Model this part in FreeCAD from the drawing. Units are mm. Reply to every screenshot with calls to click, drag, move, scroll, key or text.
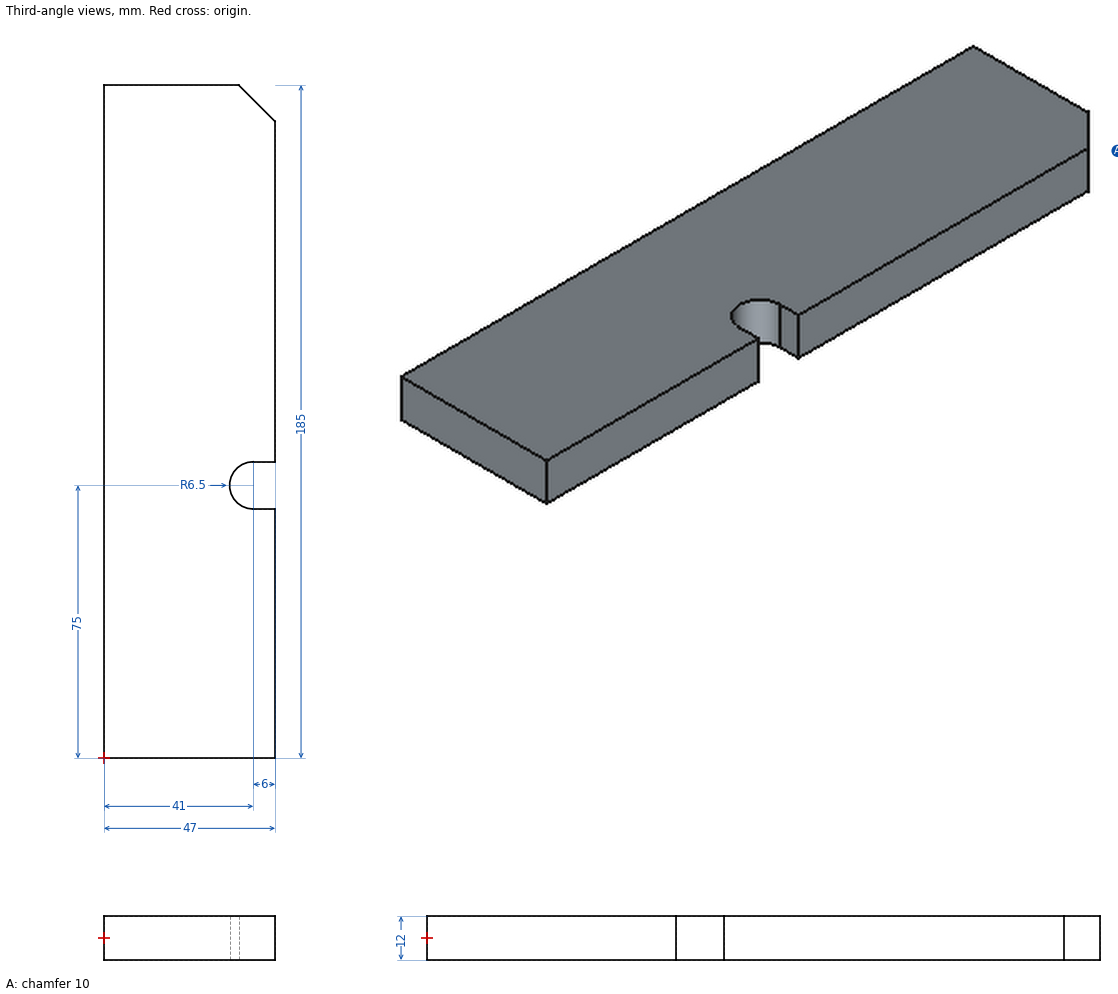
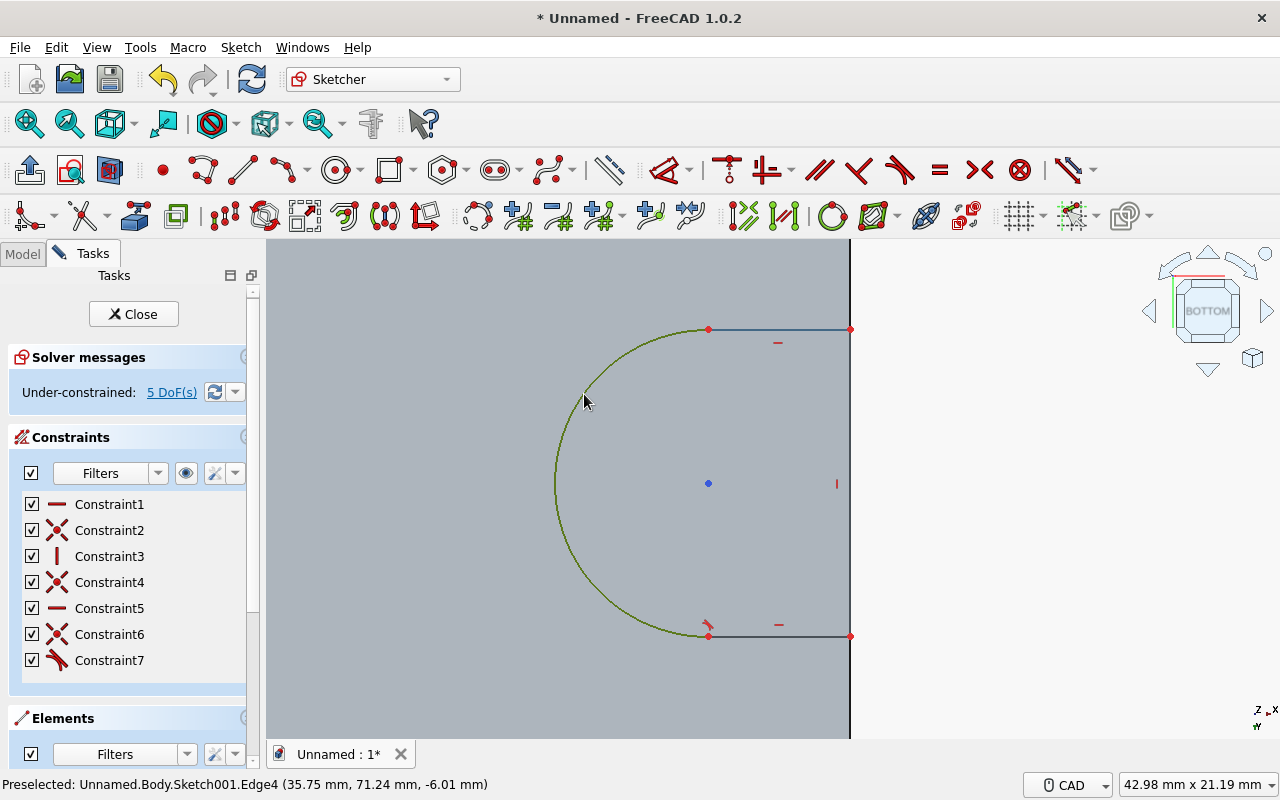
click(900, 170)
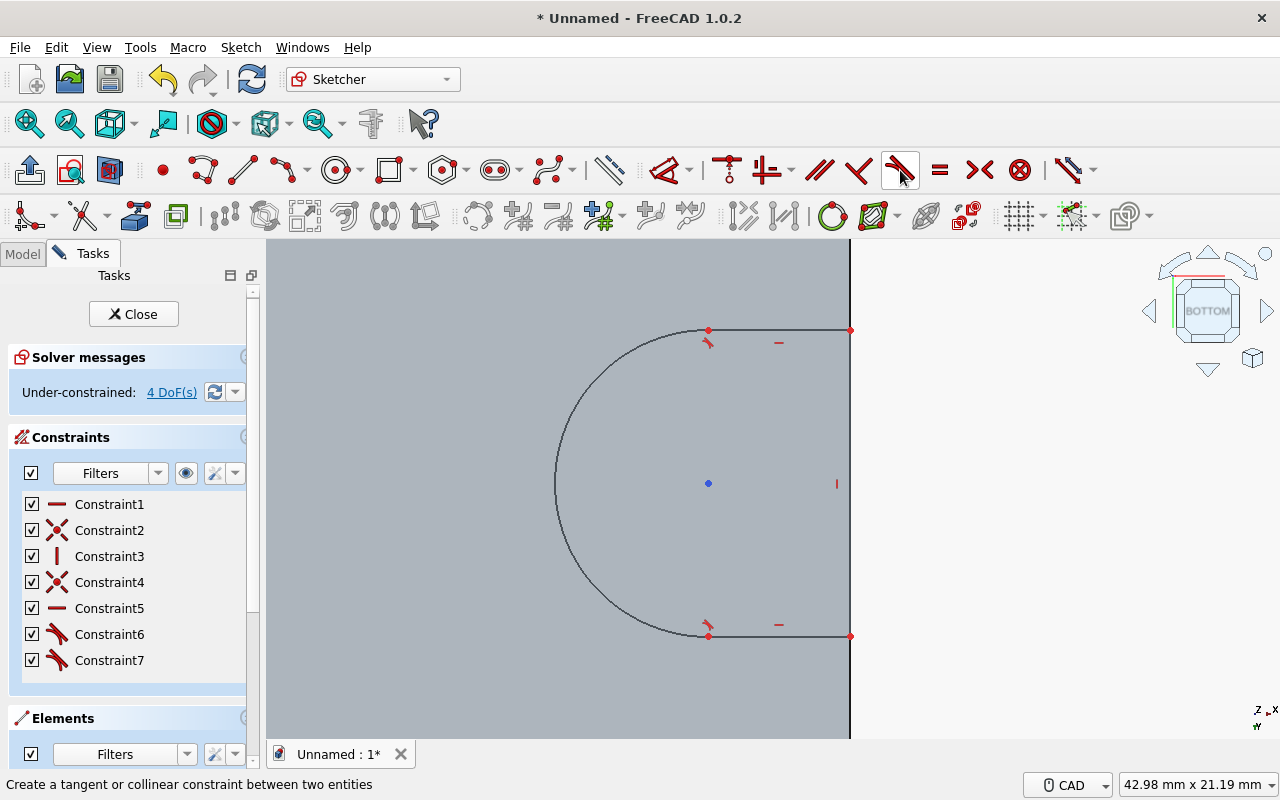
click(664, 170)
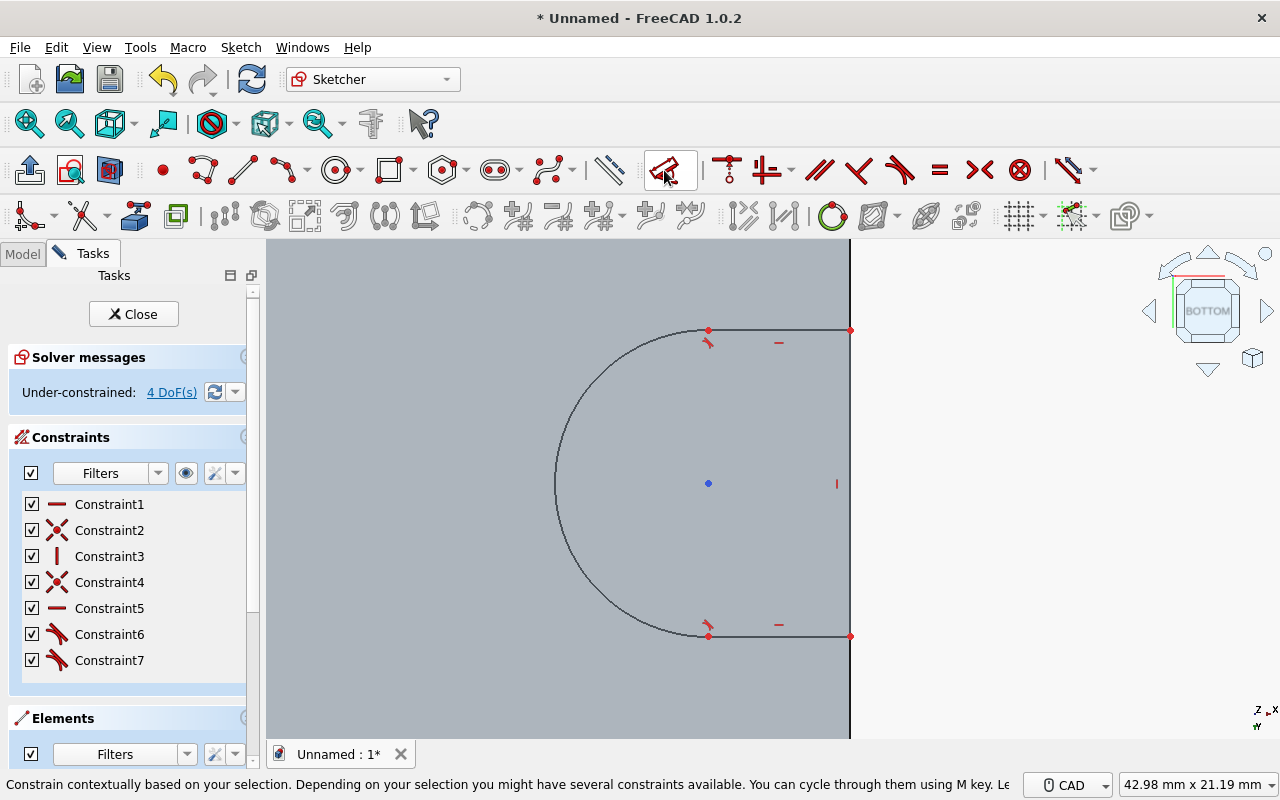
click(584, 393)
click(558, 374)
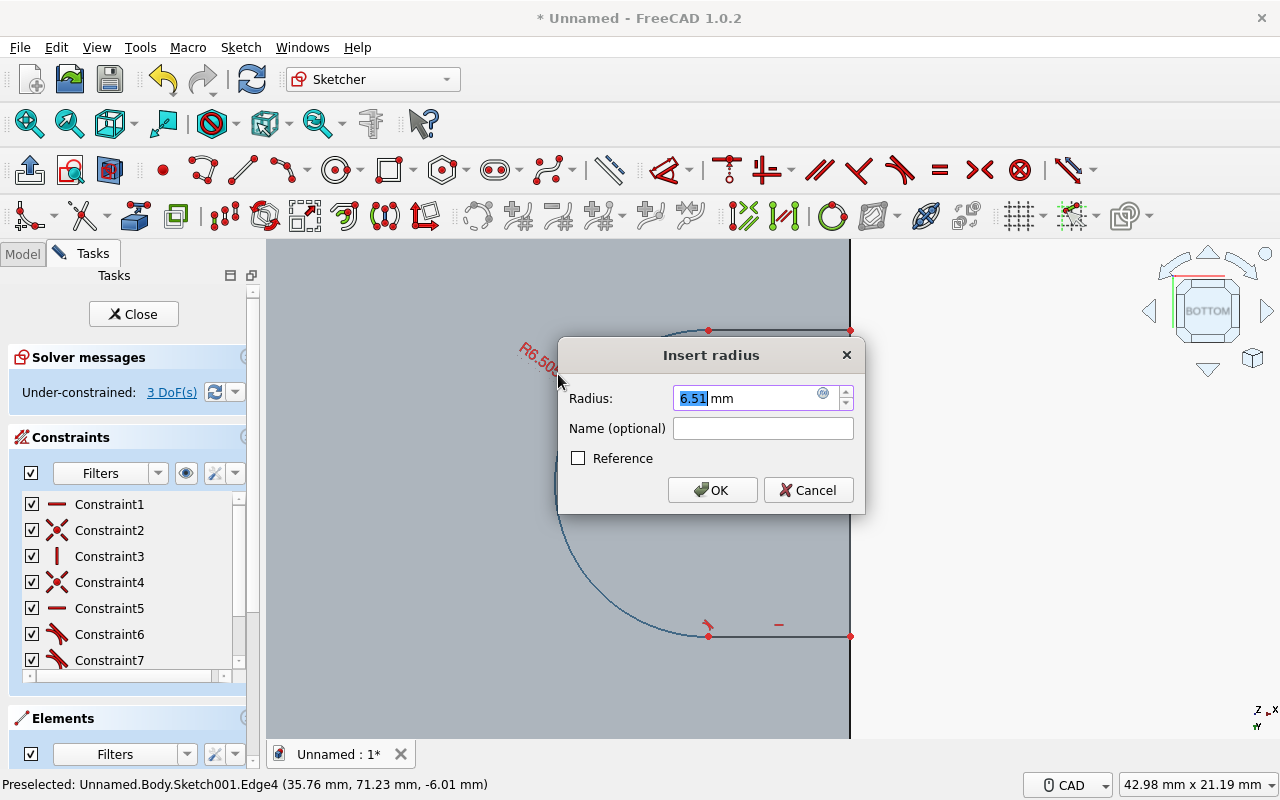
text(6.5)
key(Return)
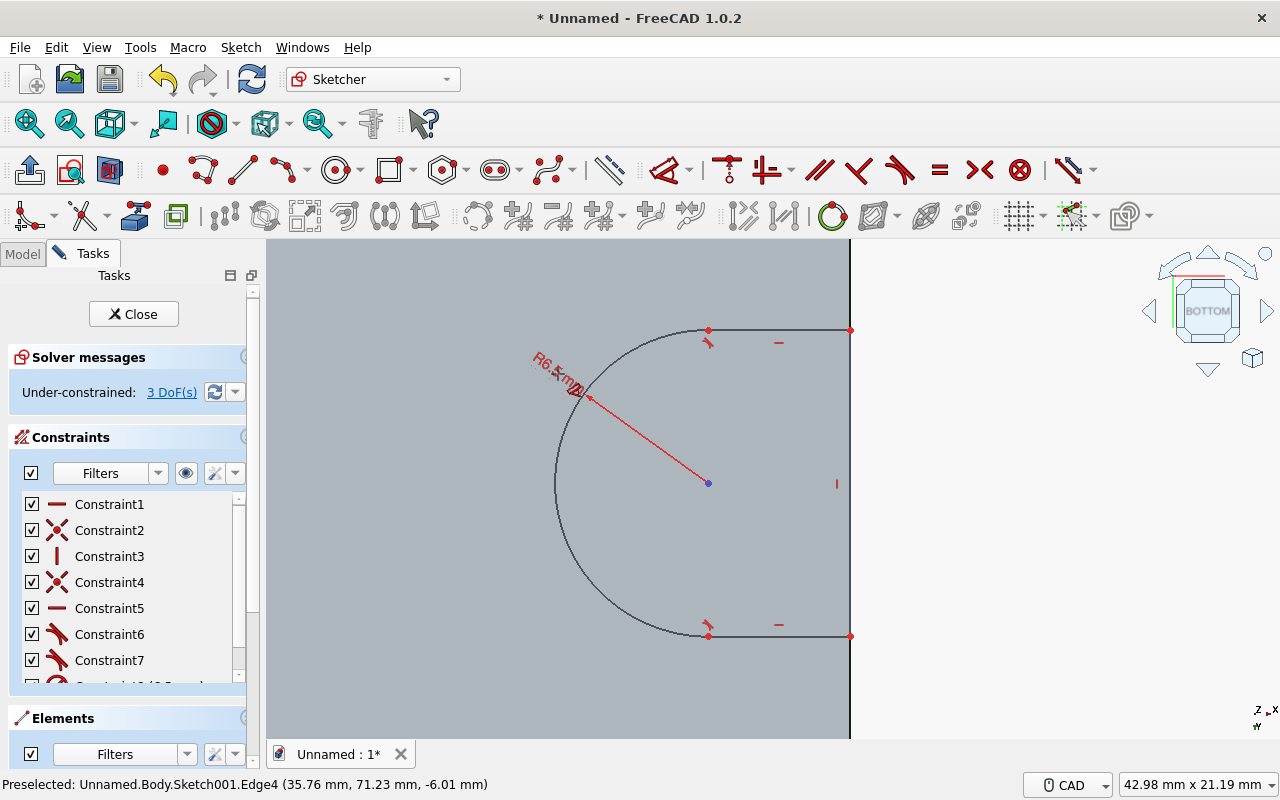
click(751, 637)
click(779, 671)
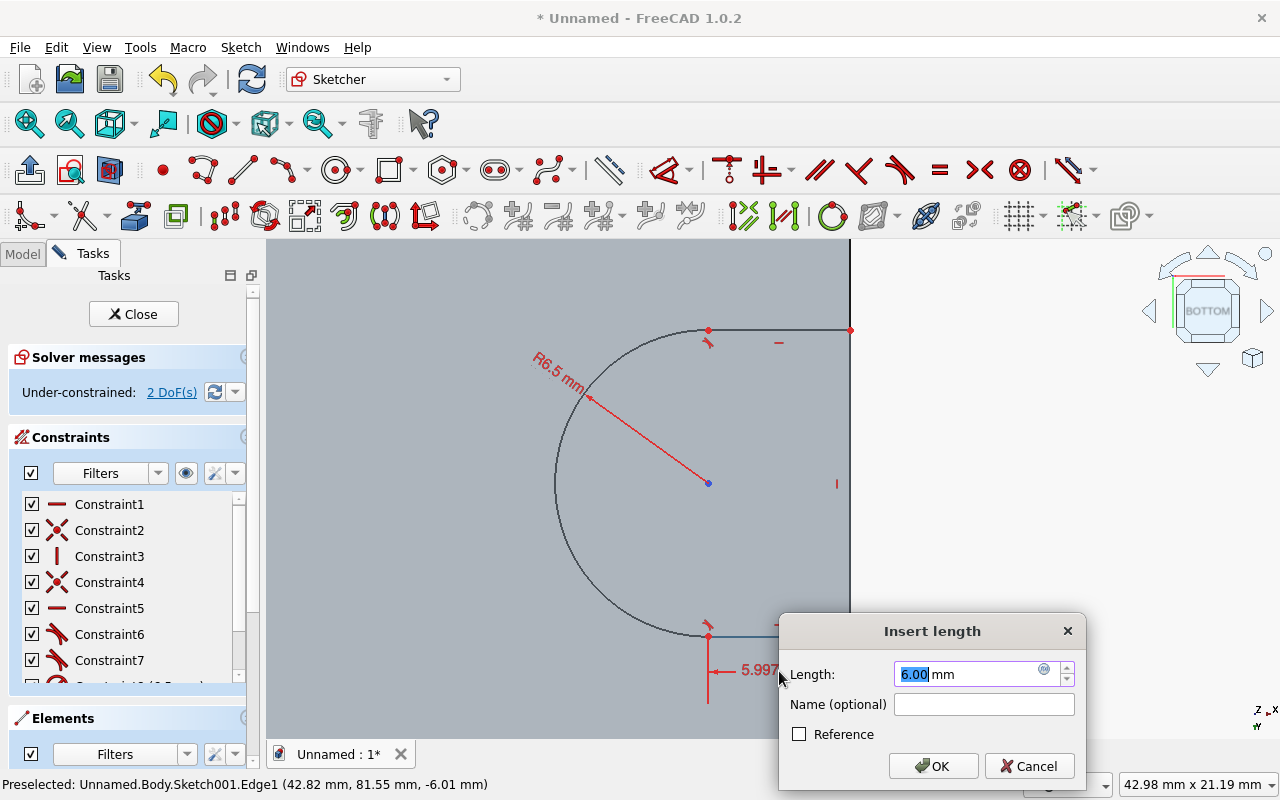
text(6)
key(Return)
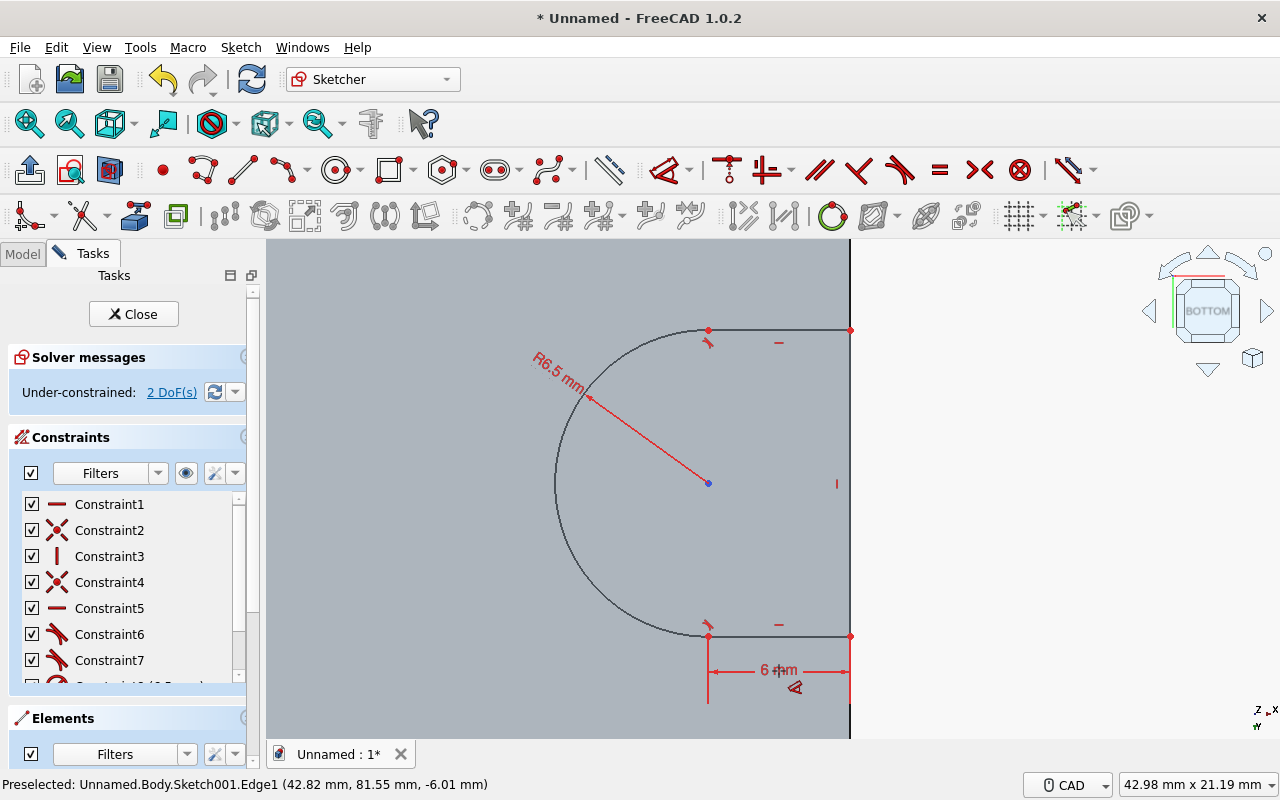
click(708, 637)
click(501, 671)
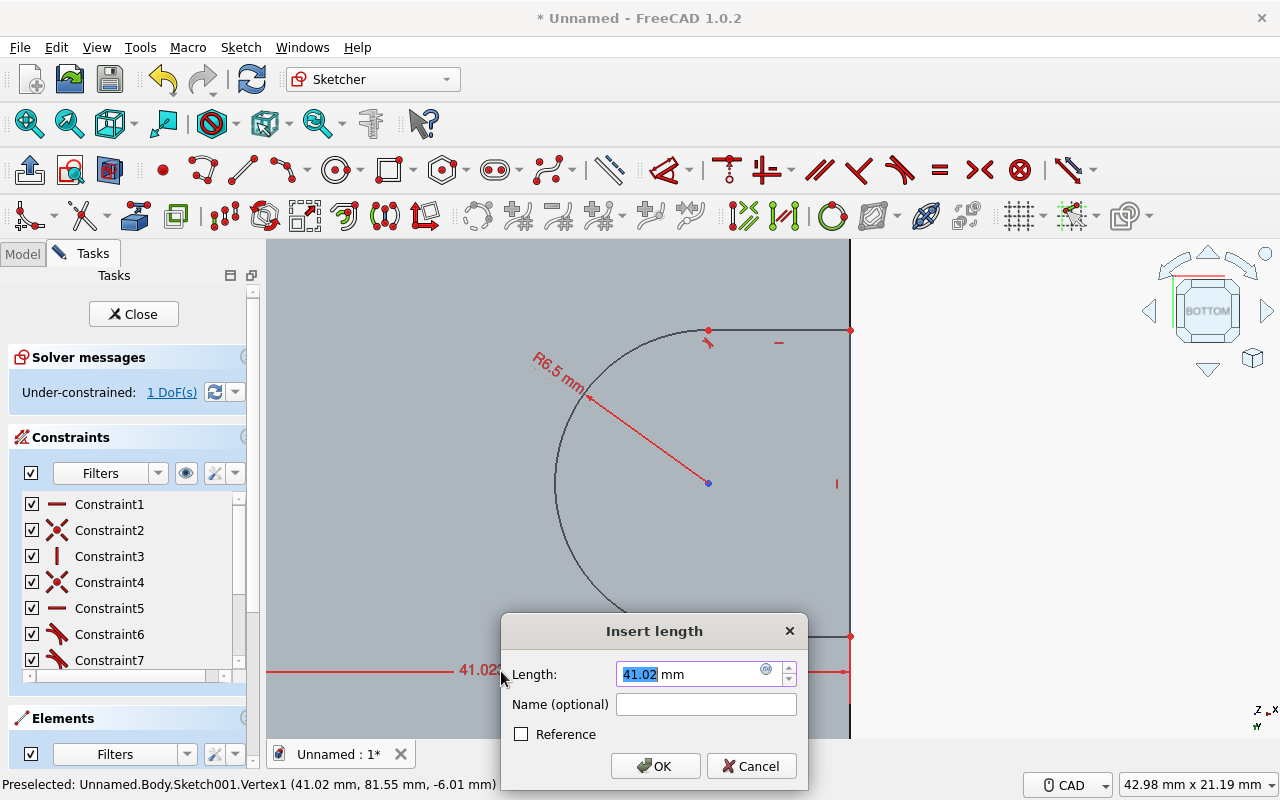
text(41)
key(Return)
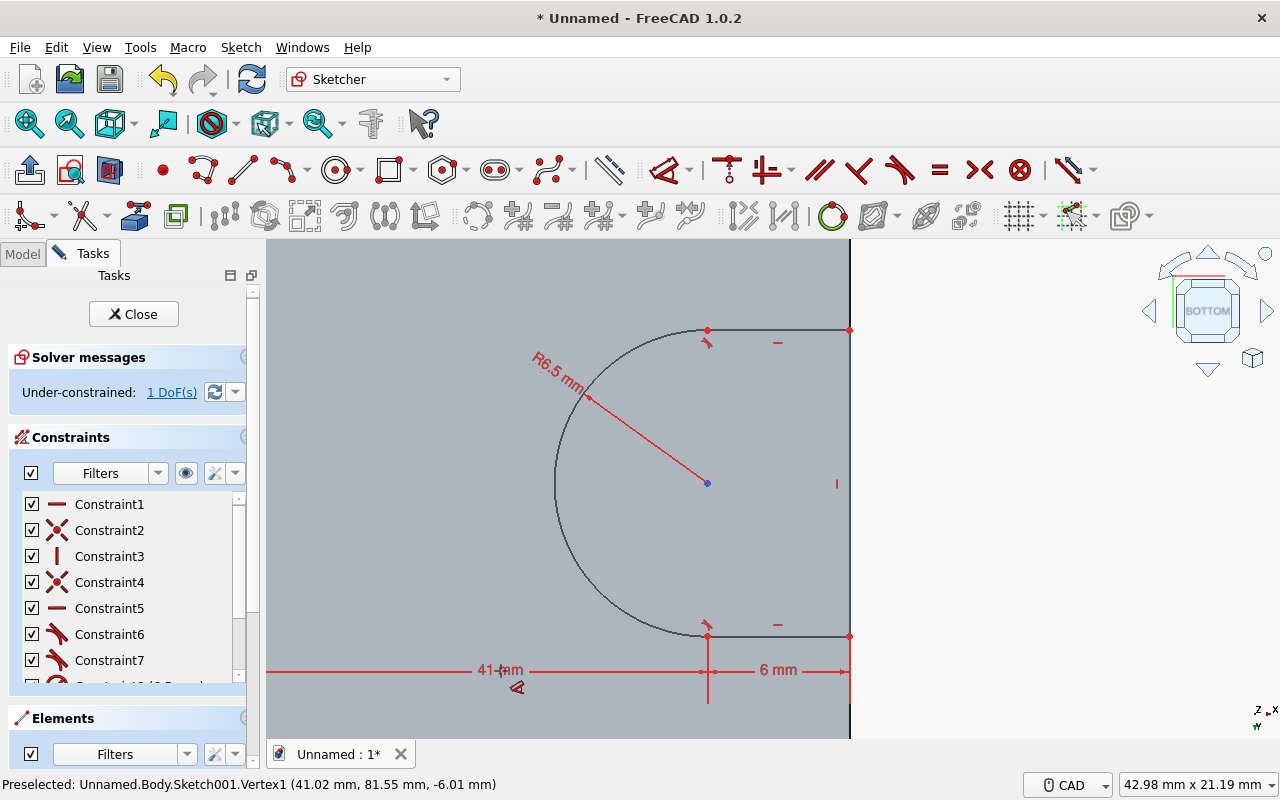
click(708, 483)
click(742, 375)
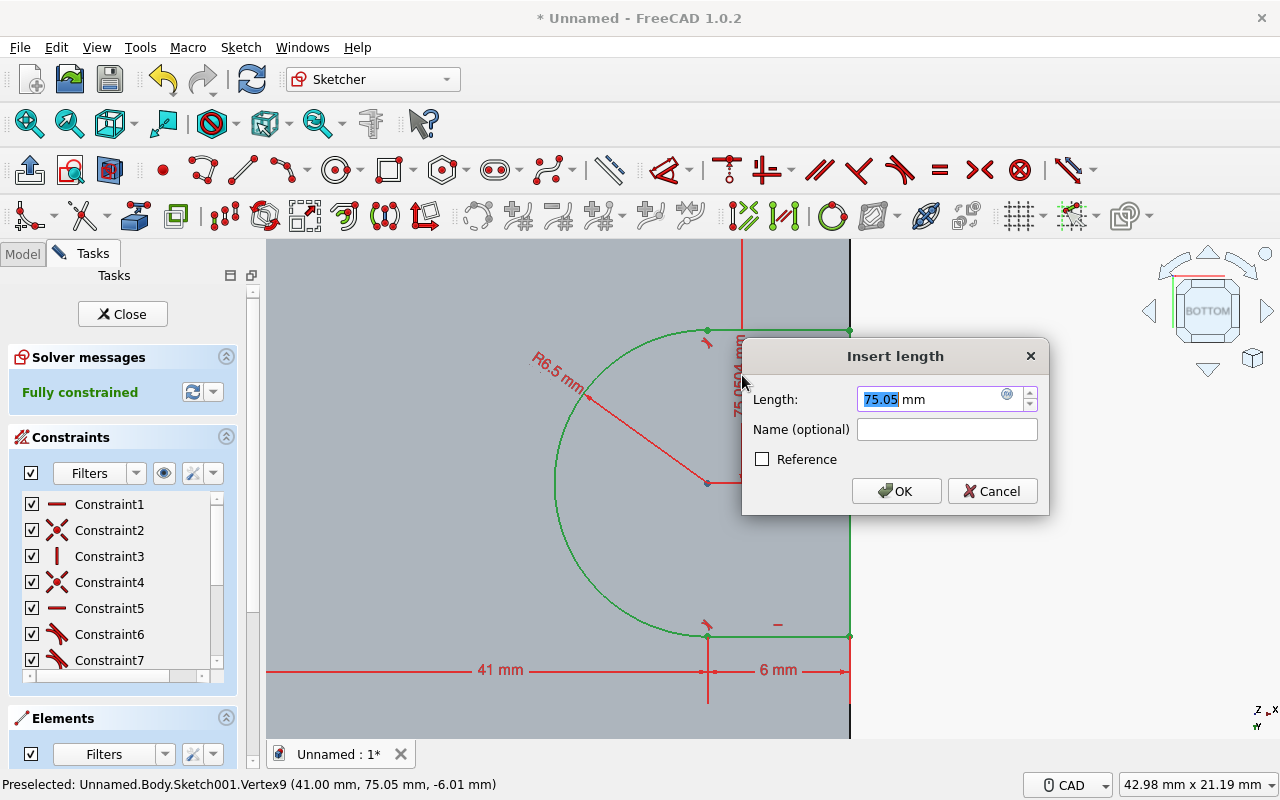
text(75)
key(Return)
key(Escape)